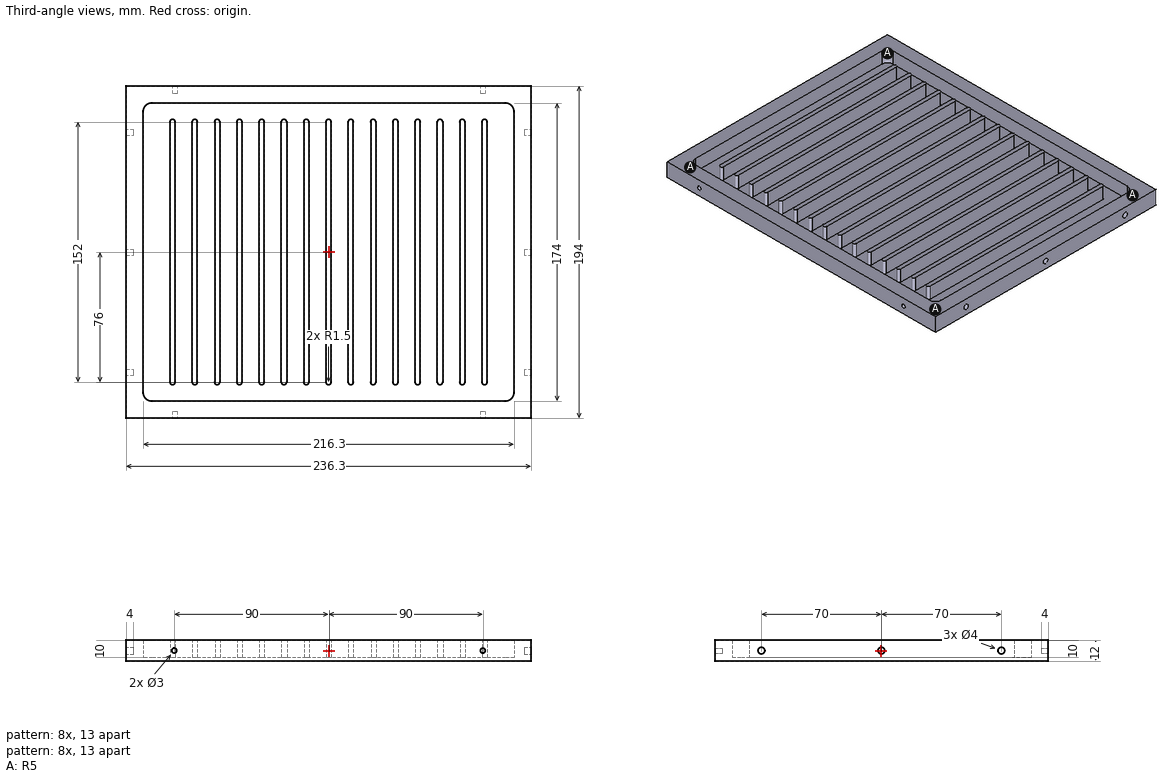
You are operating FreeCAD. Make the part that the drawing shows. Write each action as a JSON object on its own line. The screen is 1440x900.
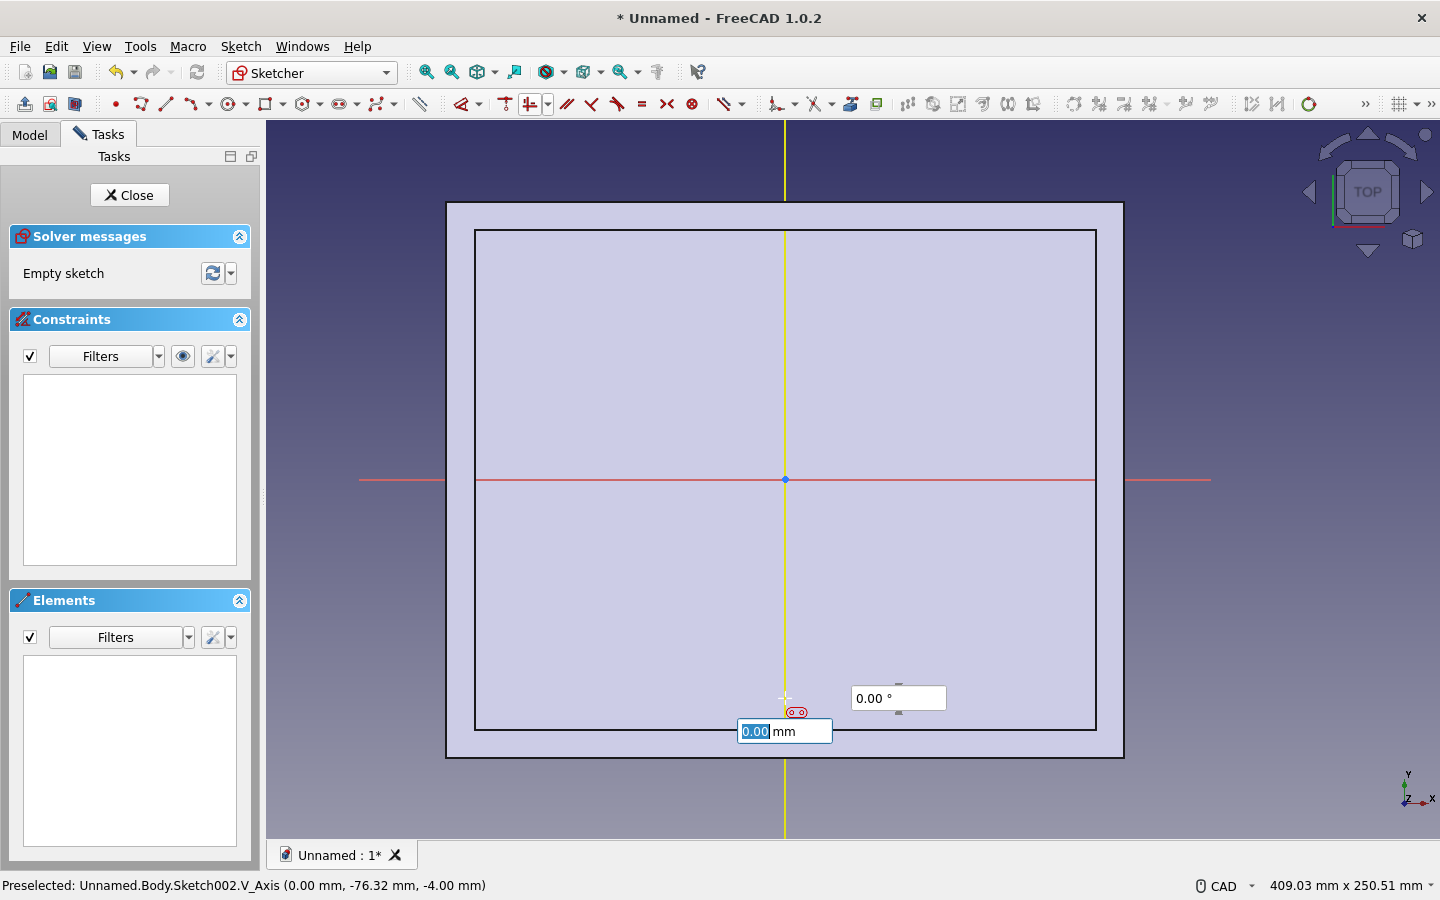
{"action": "left_click", "coordinate": [794, 262]}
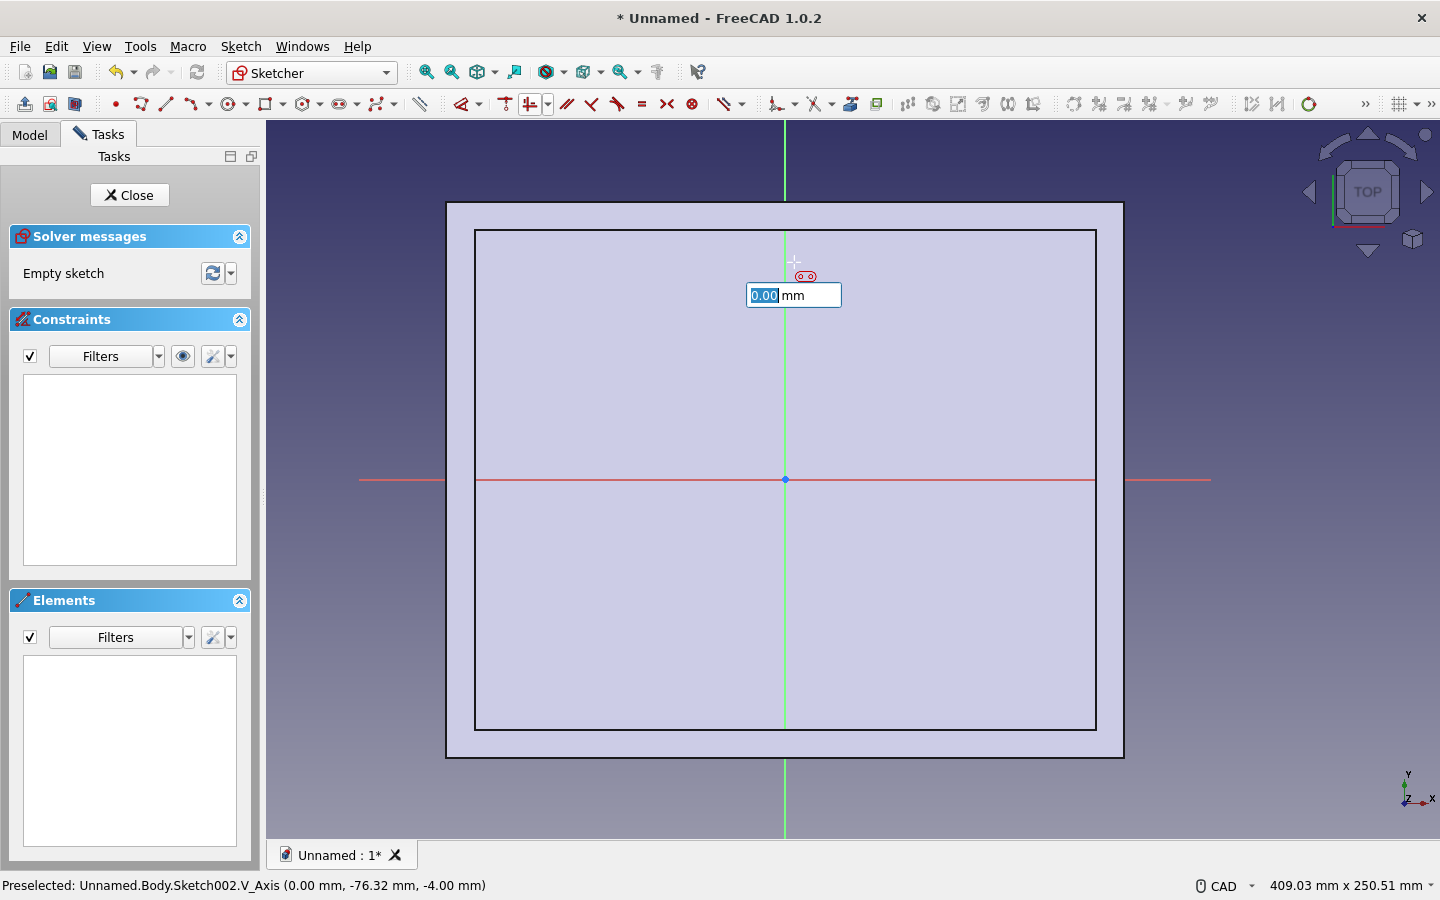
{"action": "scroll", "coordinate": [781, 414], "scroll_direction": "up", "scroll_amount": 7}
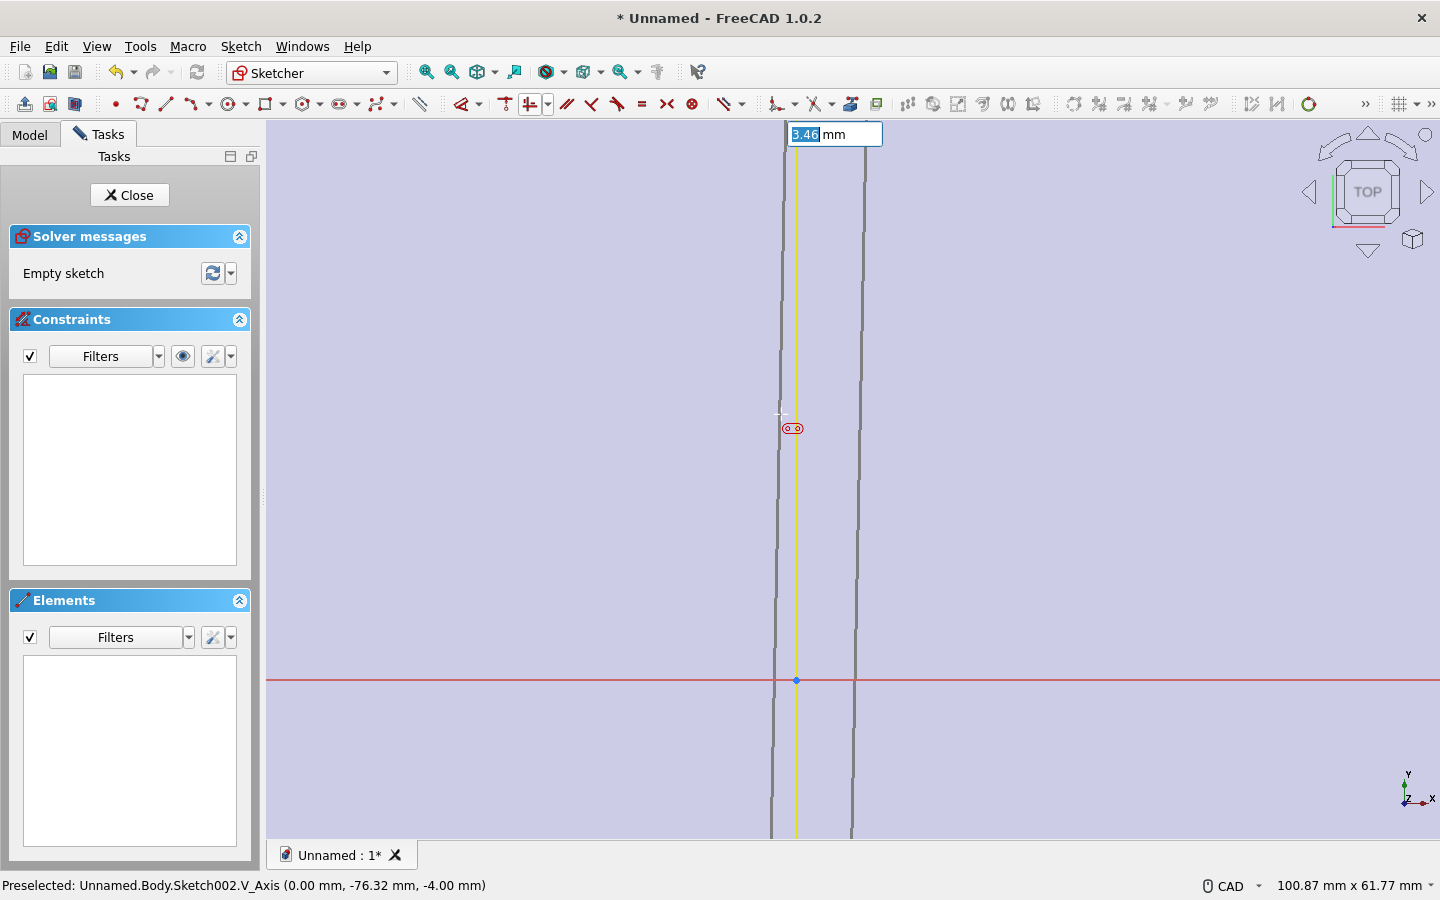
{"action": "left_click", "coordinate": [779, 415]}
{"action": "key", "text": "Escape"}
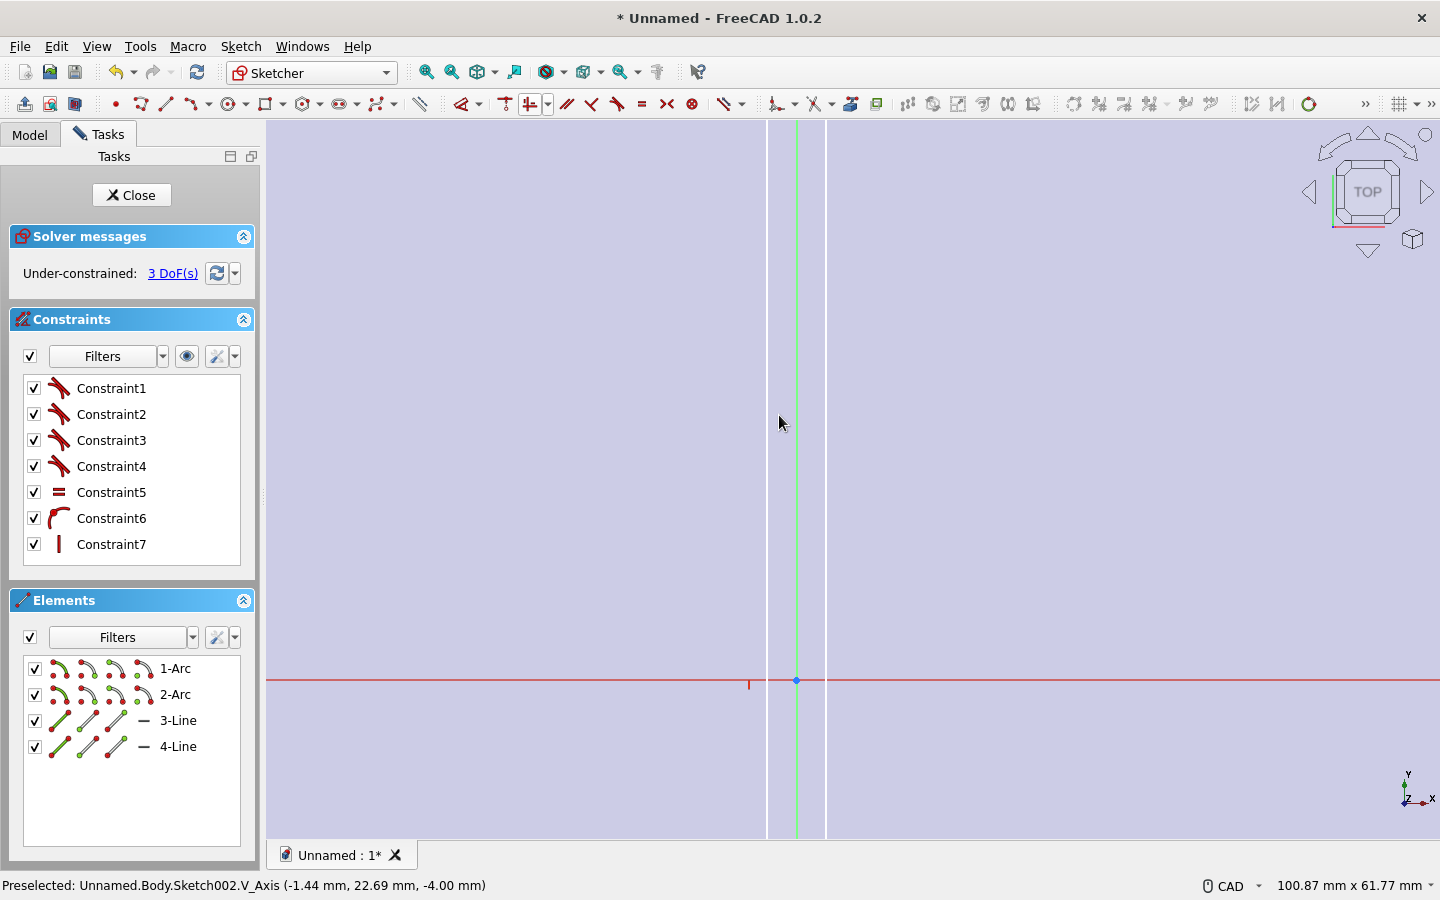
{"action": "left_click", "coordinate": [460, 104]}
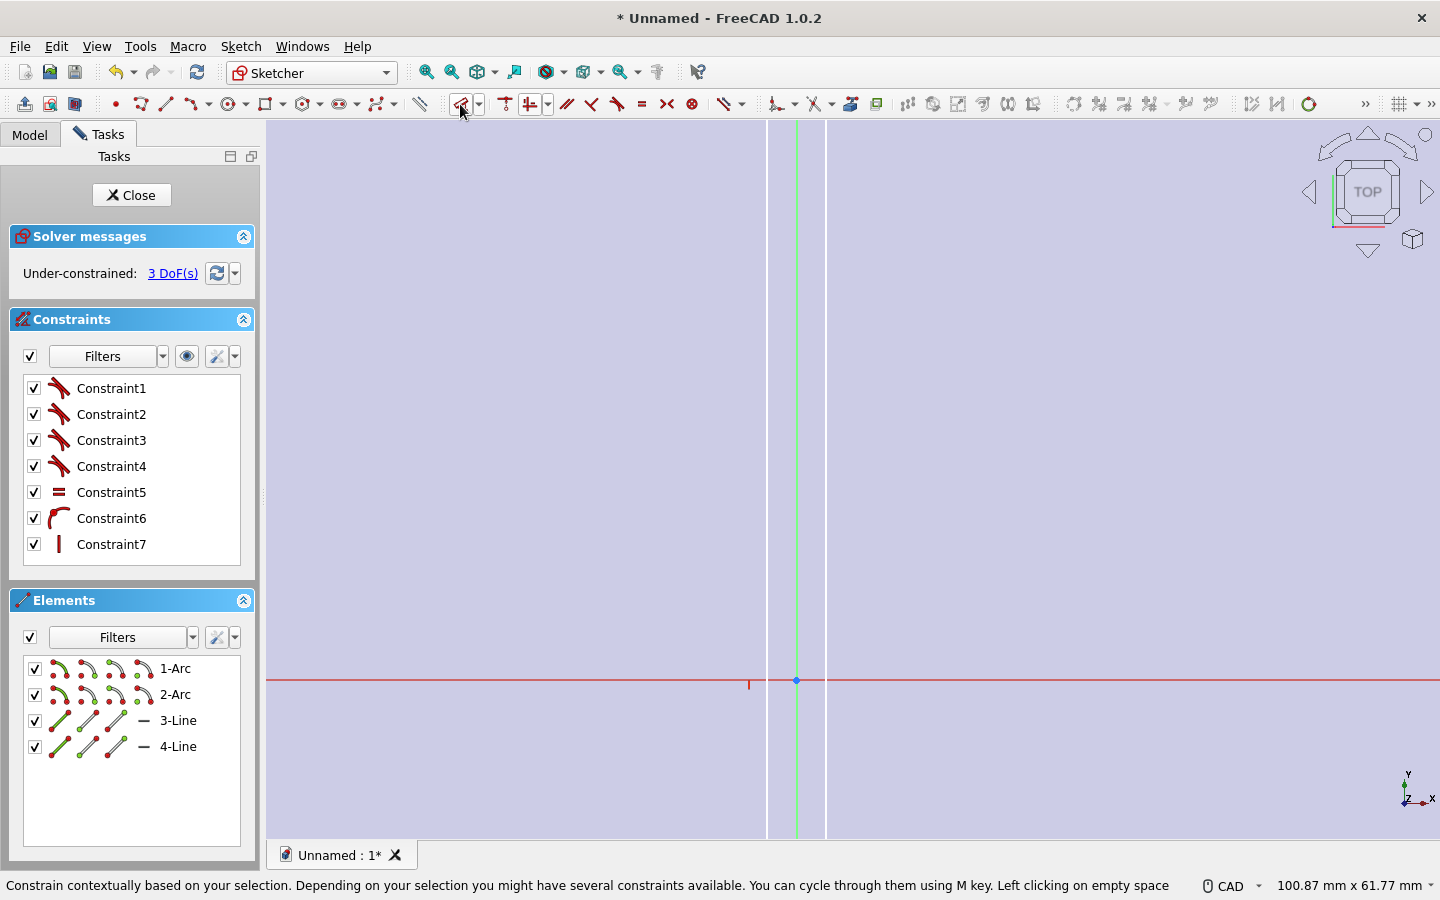
{"action": "scroll", "coordinate": [780, 414], "scroll_direction": "down", "scroll_amount": 7}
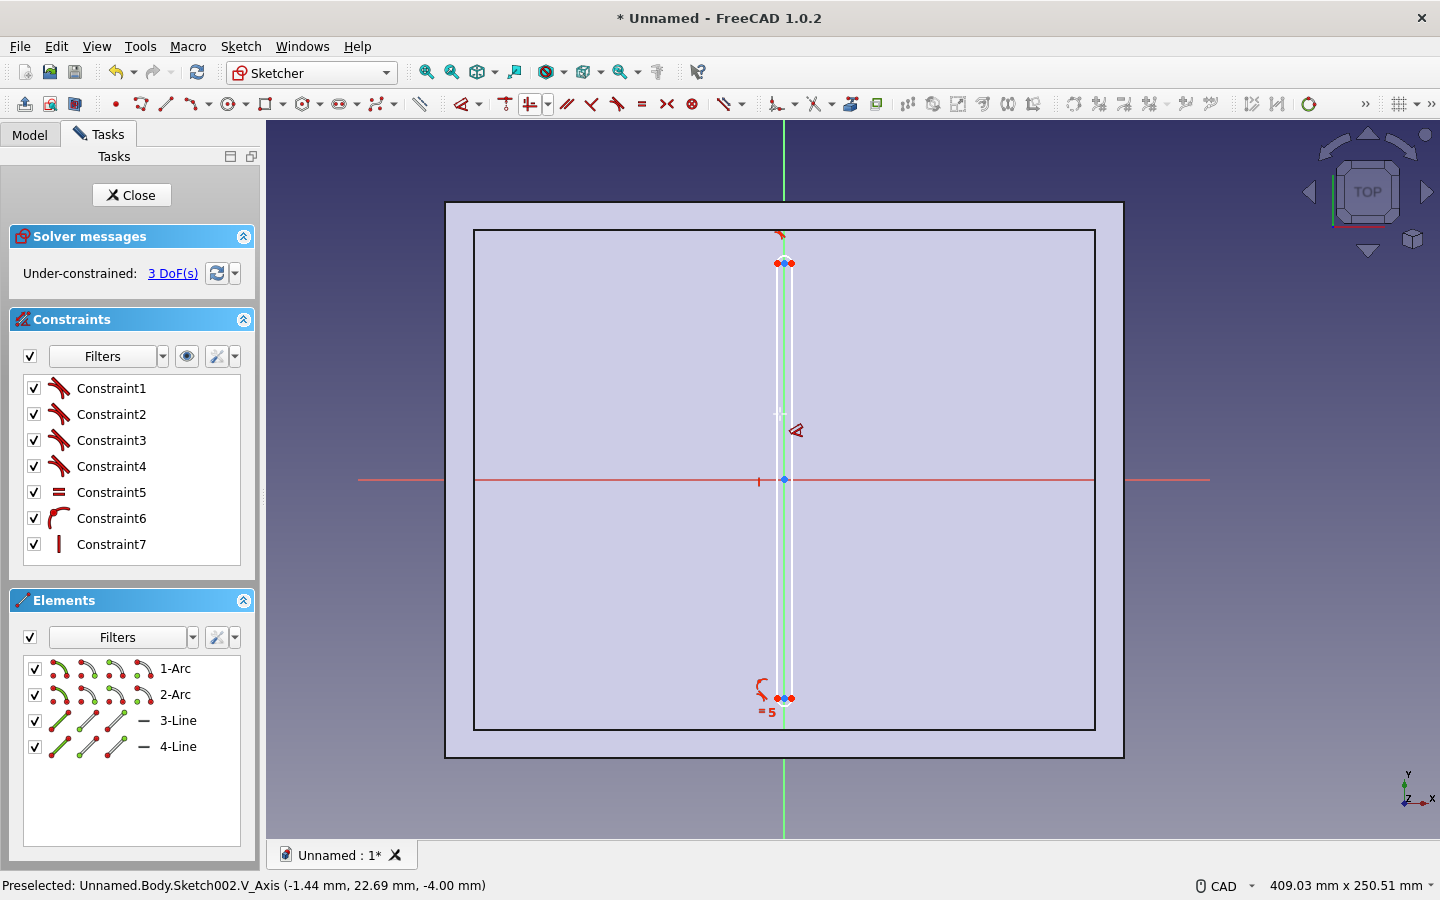
{"action": "scroll", "coordinate": [780, 705], "scroll_direction": "up", "scroll_amount": 12}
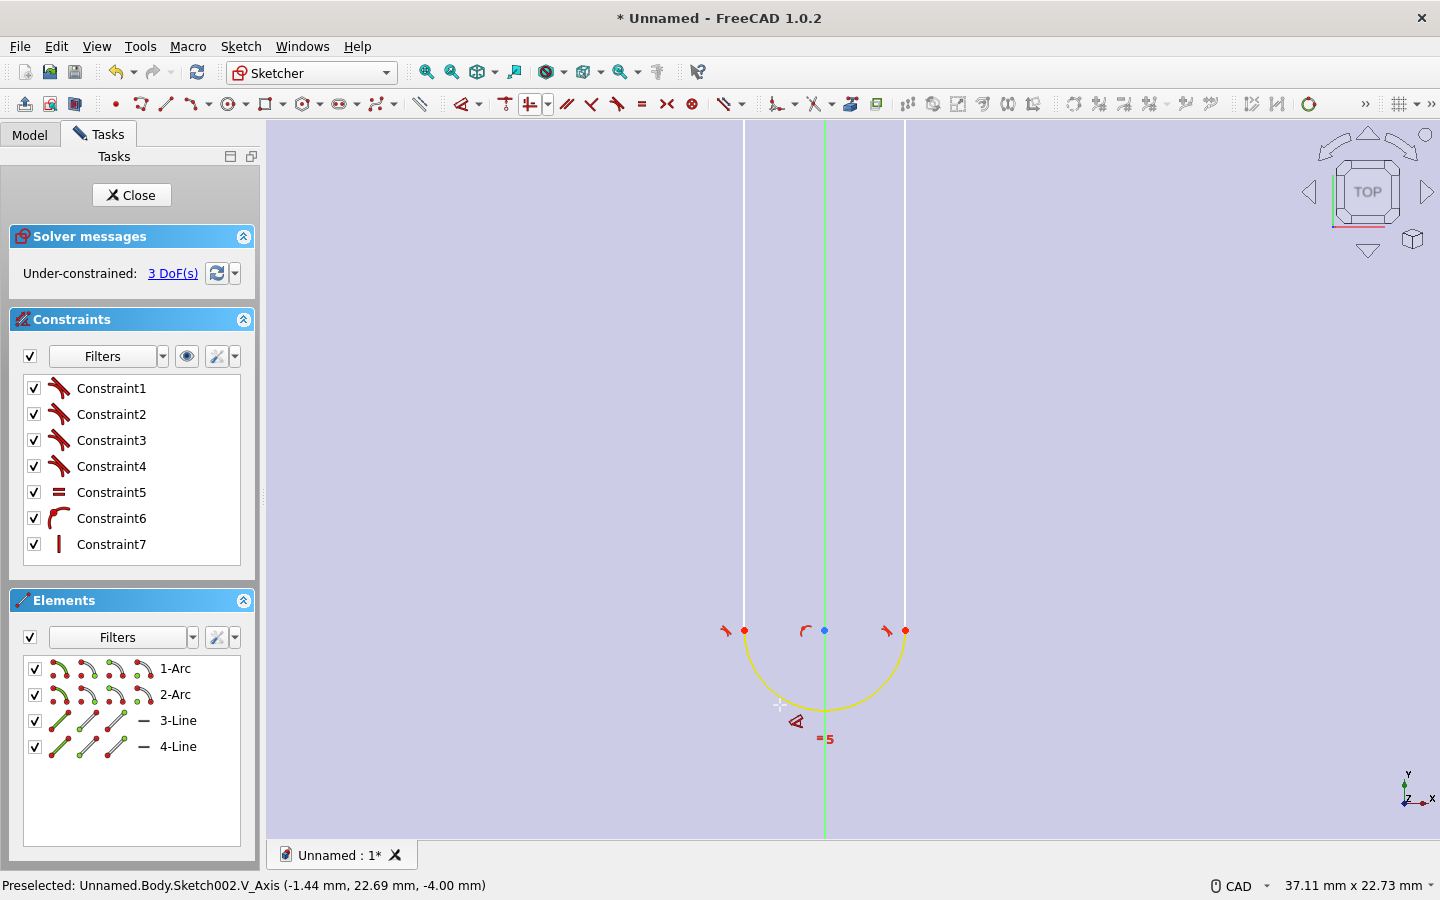
{"action": "left_click", "coordinate": [778, 695]}
{"action": "left_click", "coordinate": [759, 721]}